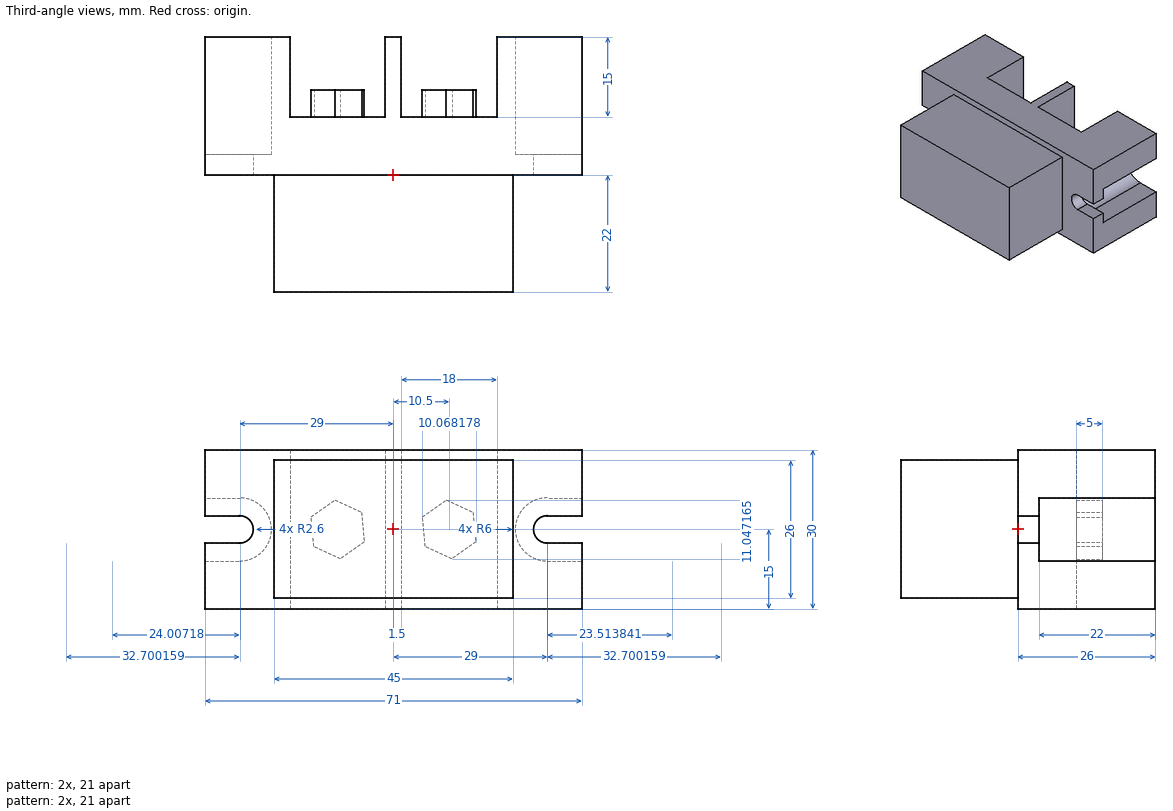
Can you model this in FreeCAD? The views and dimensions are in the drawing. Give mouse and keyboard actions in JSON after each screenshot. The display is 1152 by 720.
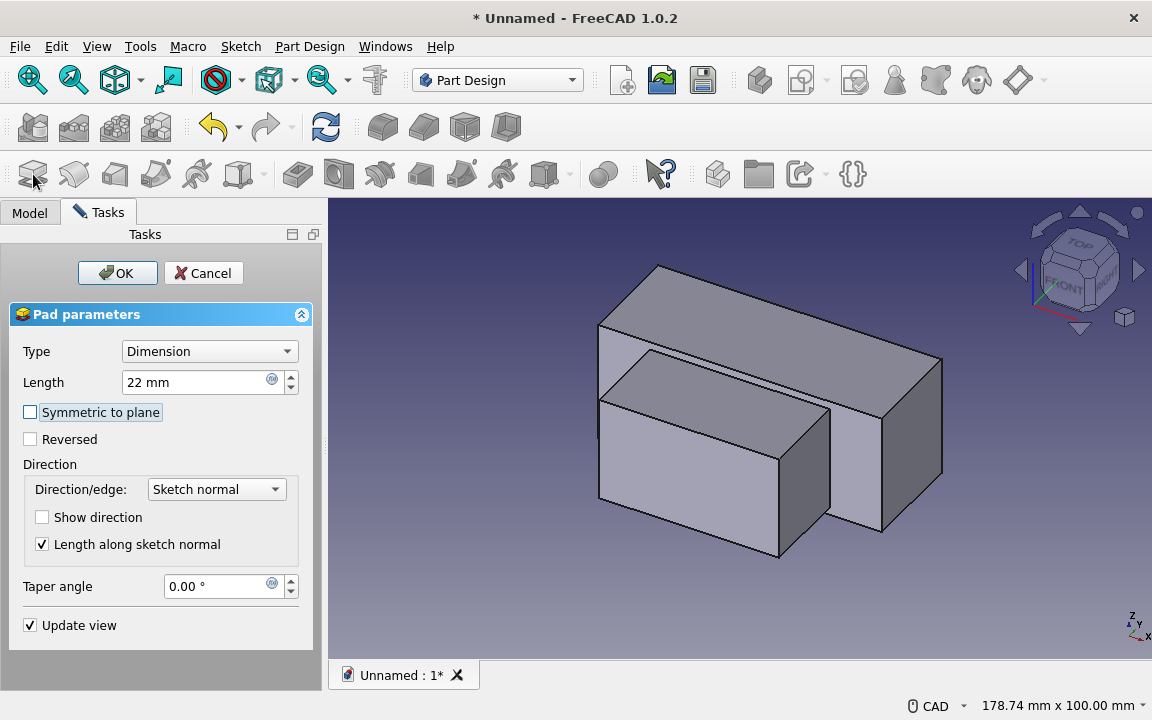
{"action": "left_click", "coordinate": [118, 273]}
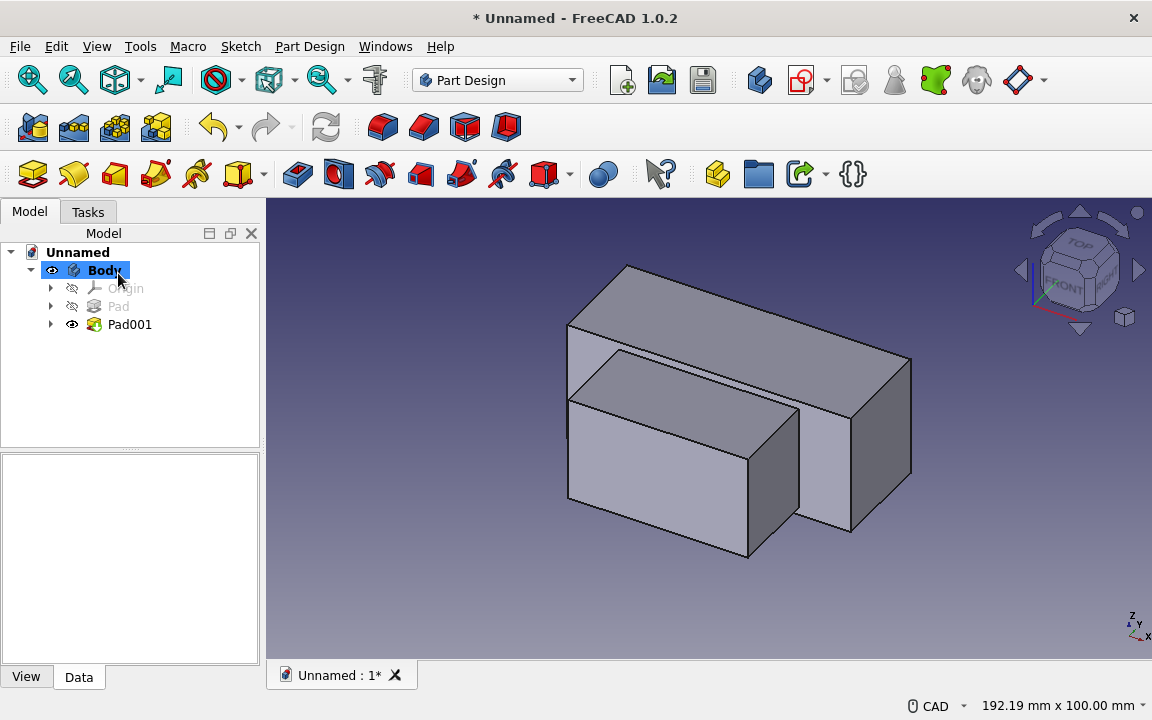
{"action": "key", "text": "4"}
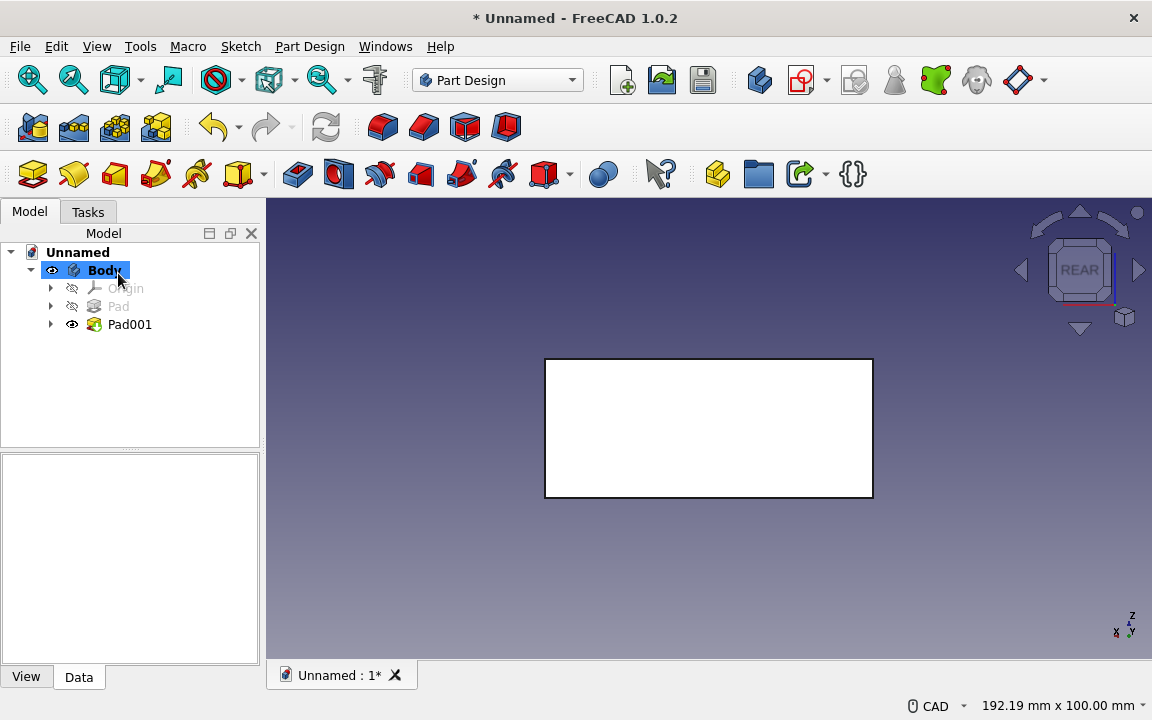
{"action": "key", "text": "v f"}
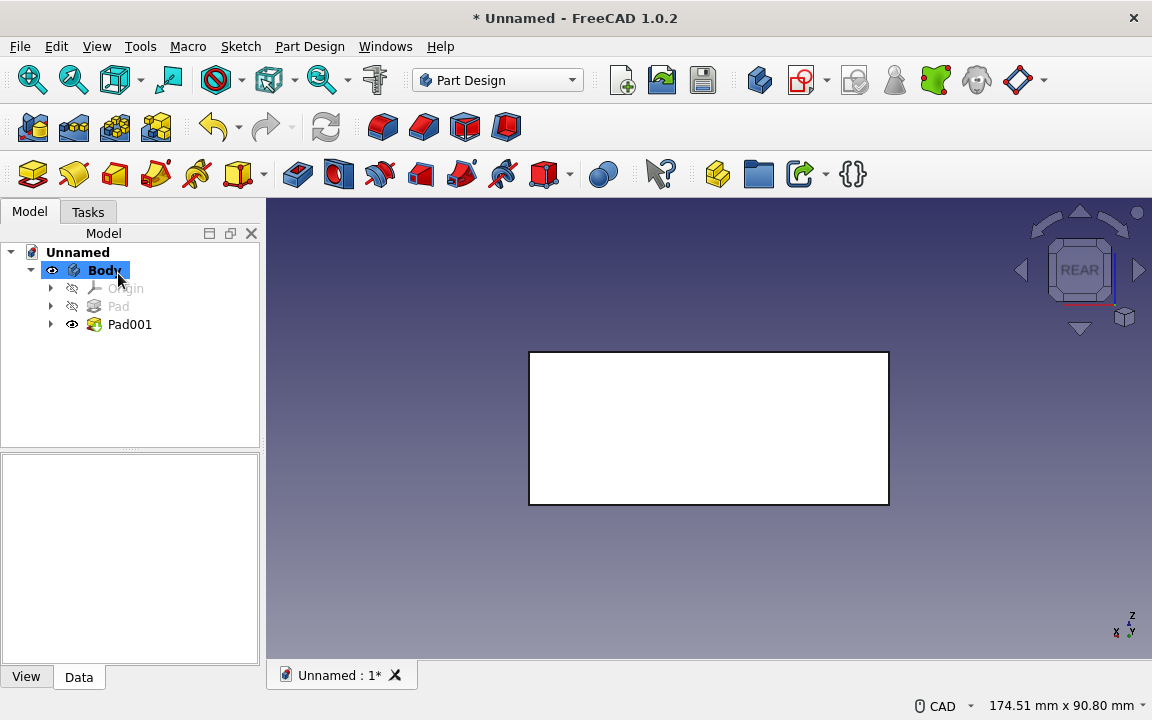
{"action": "left_click", "coordinate": [606, 428]}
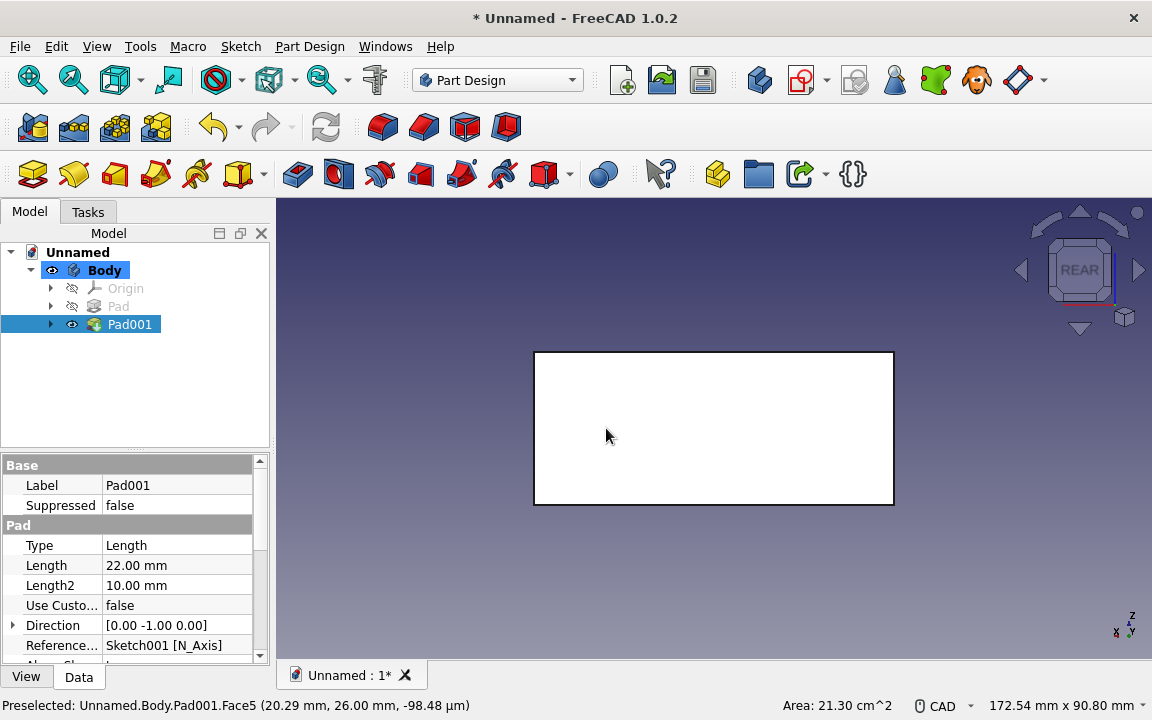
{"action": "left_click", "coordinate": [800, 80]}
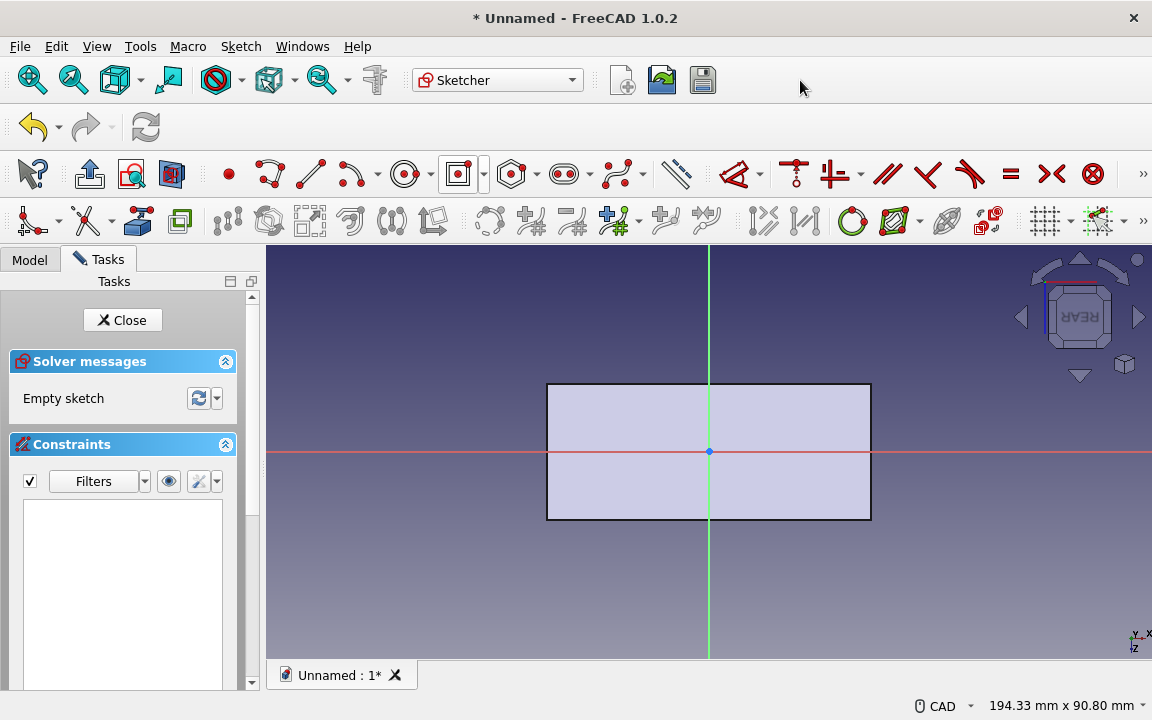
{"action": "scroll", "coordinate": [331, 452], "scroll_direction": "down", "scroll_amount": 1}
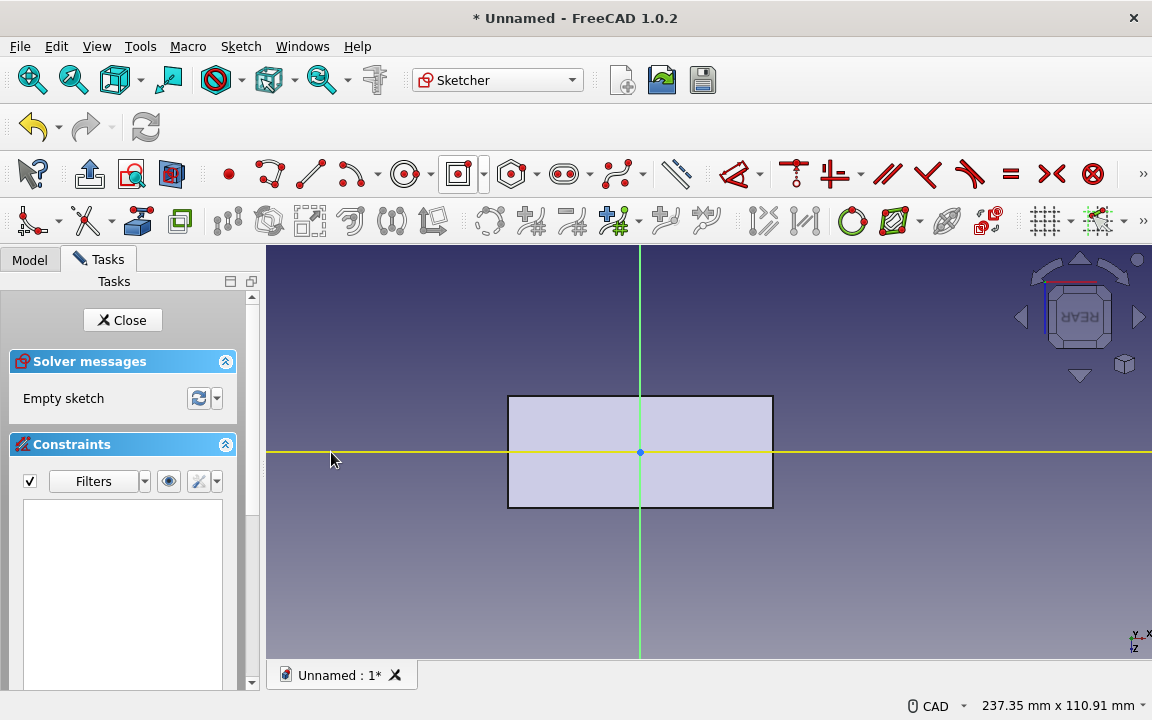
{"action": "left_click", "coordinate": [564, 174]}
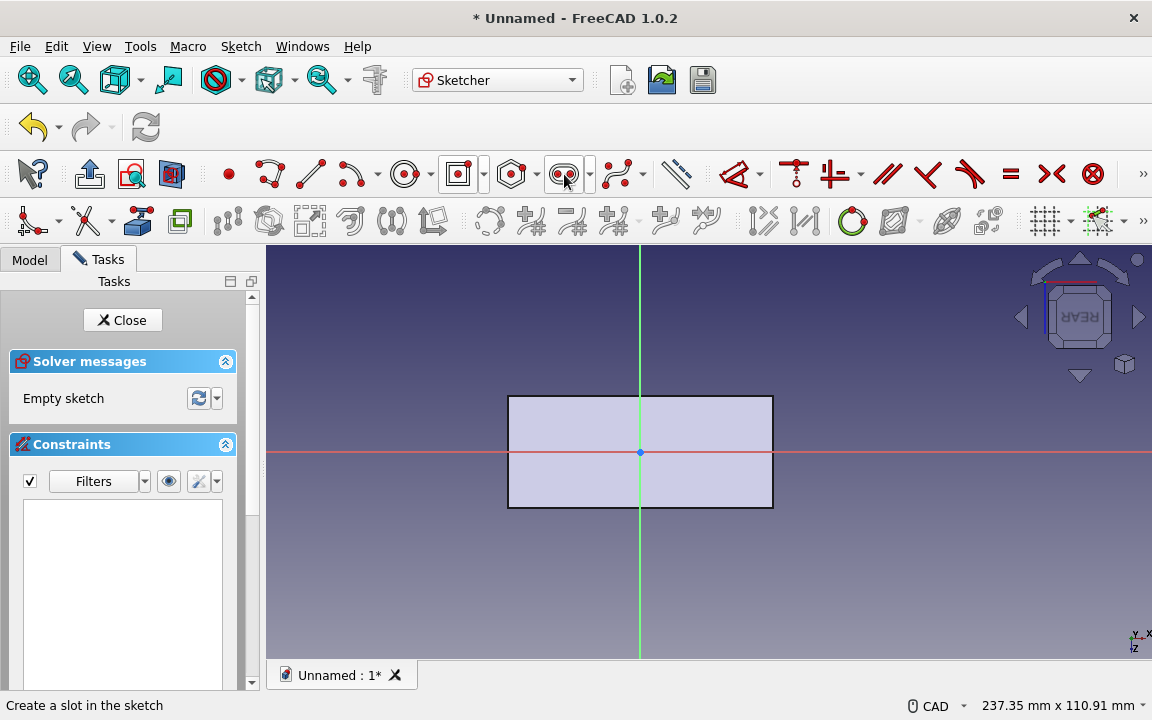
{"action": "scroll", "coordinate": [410, 452], "scroll_direction": "up", "scroll_amount": 5}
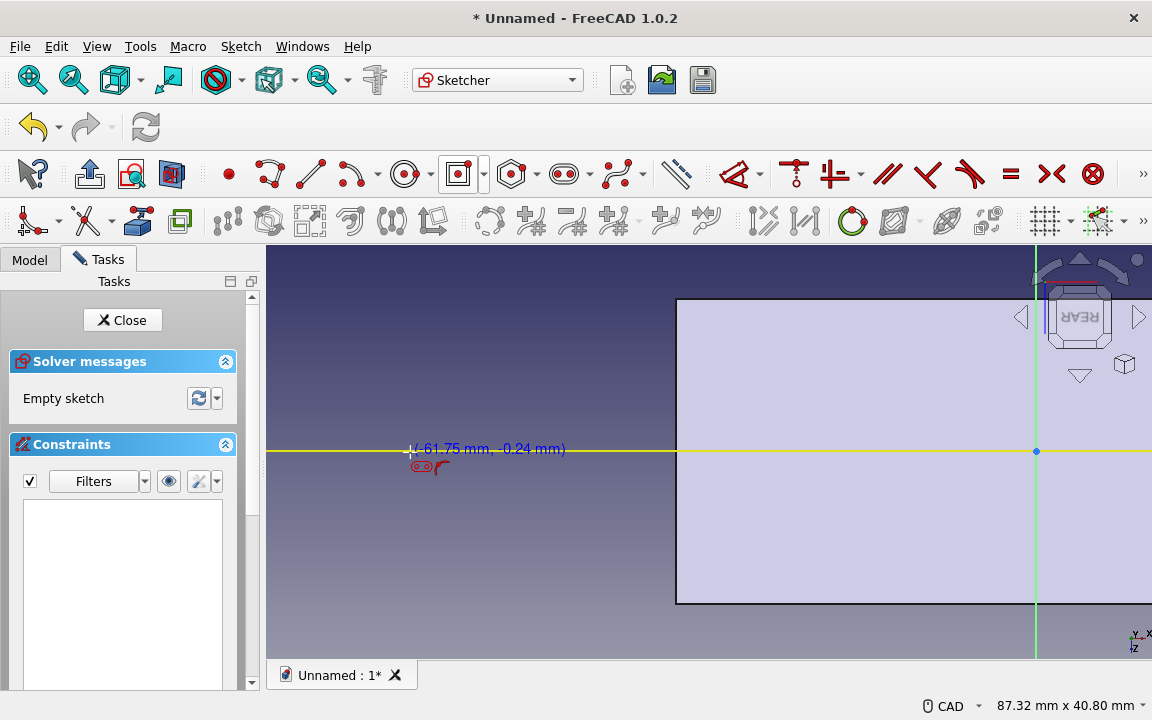
{"action": "left_click", "coordinate": [410, 451]}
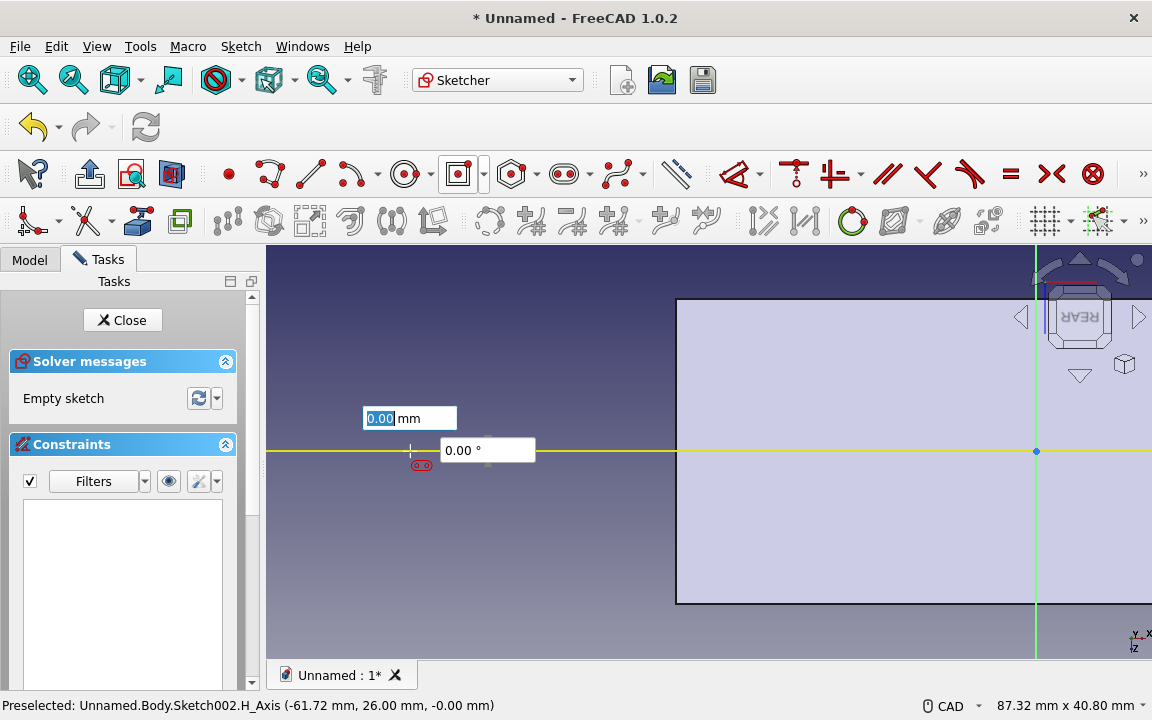
{"action": "left_click", "coordinate": [742, 442]}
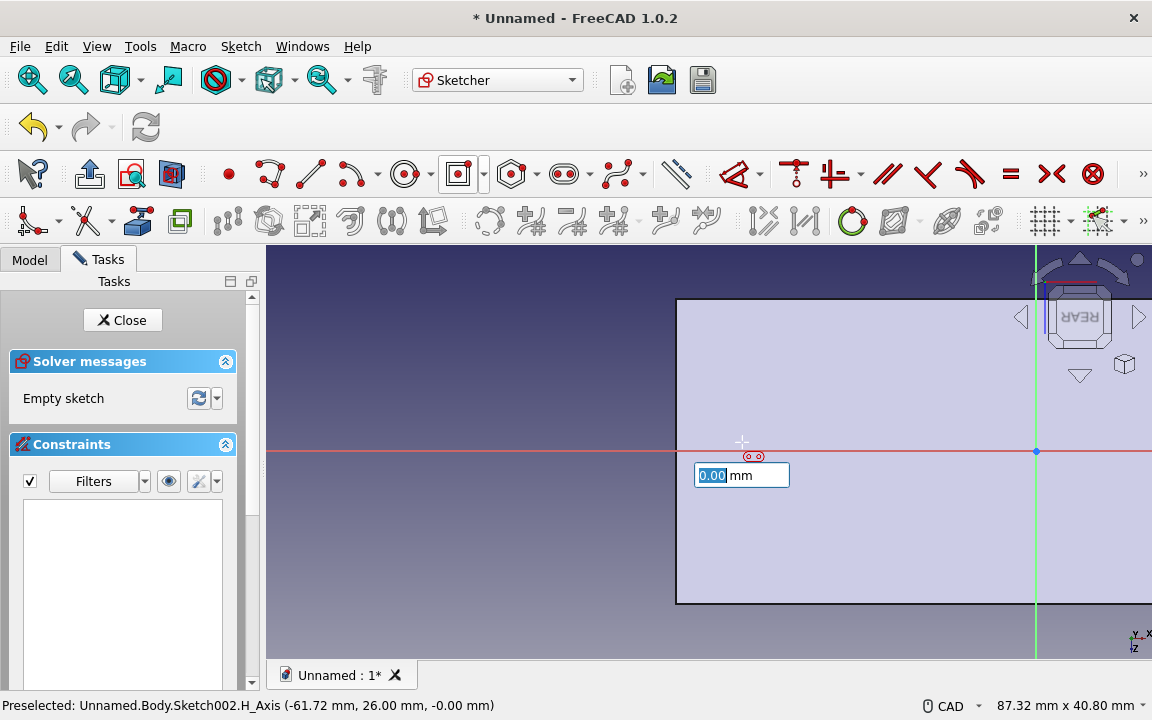
{"action": "left_click", "coordinate": [576, 478]}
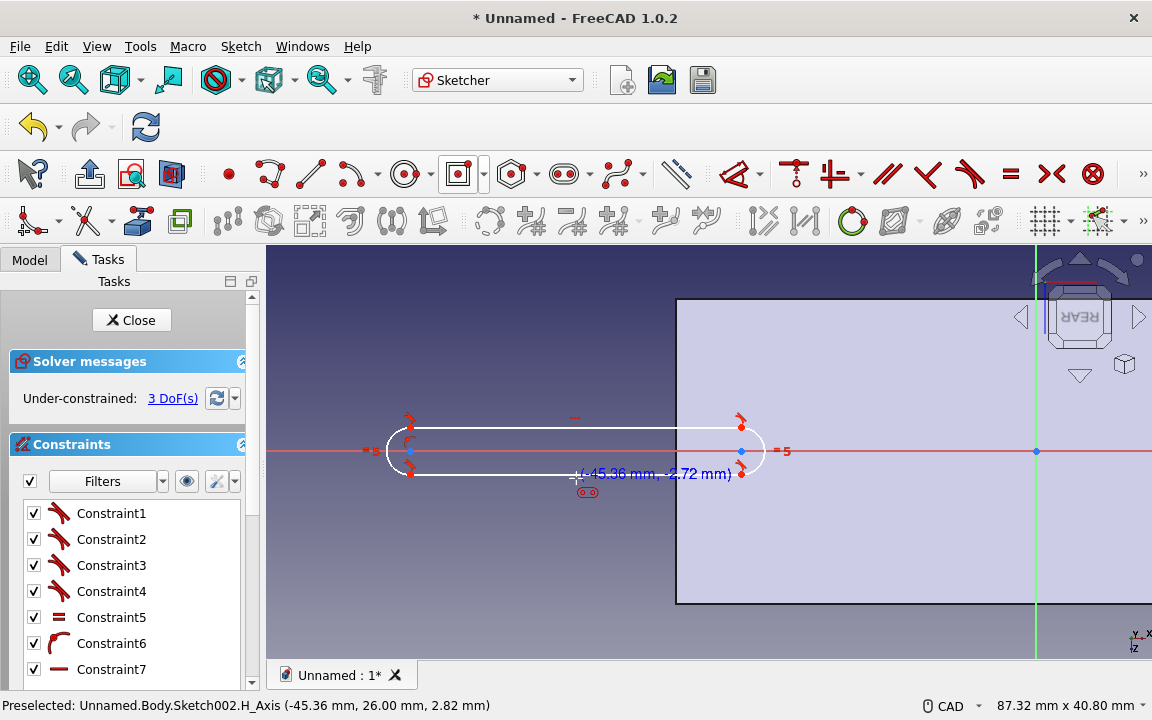
{"action": "scroll", "coordinate": [410, 452], "scroll_direction": "down", "scroll_amount": 5}